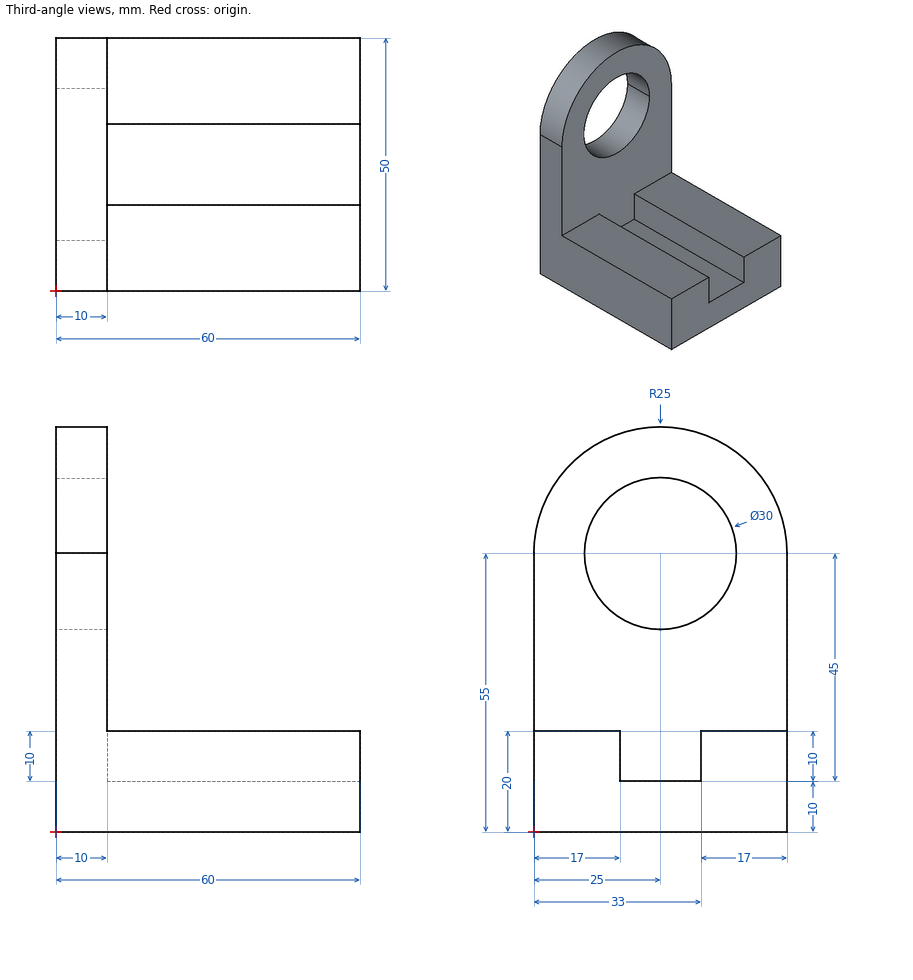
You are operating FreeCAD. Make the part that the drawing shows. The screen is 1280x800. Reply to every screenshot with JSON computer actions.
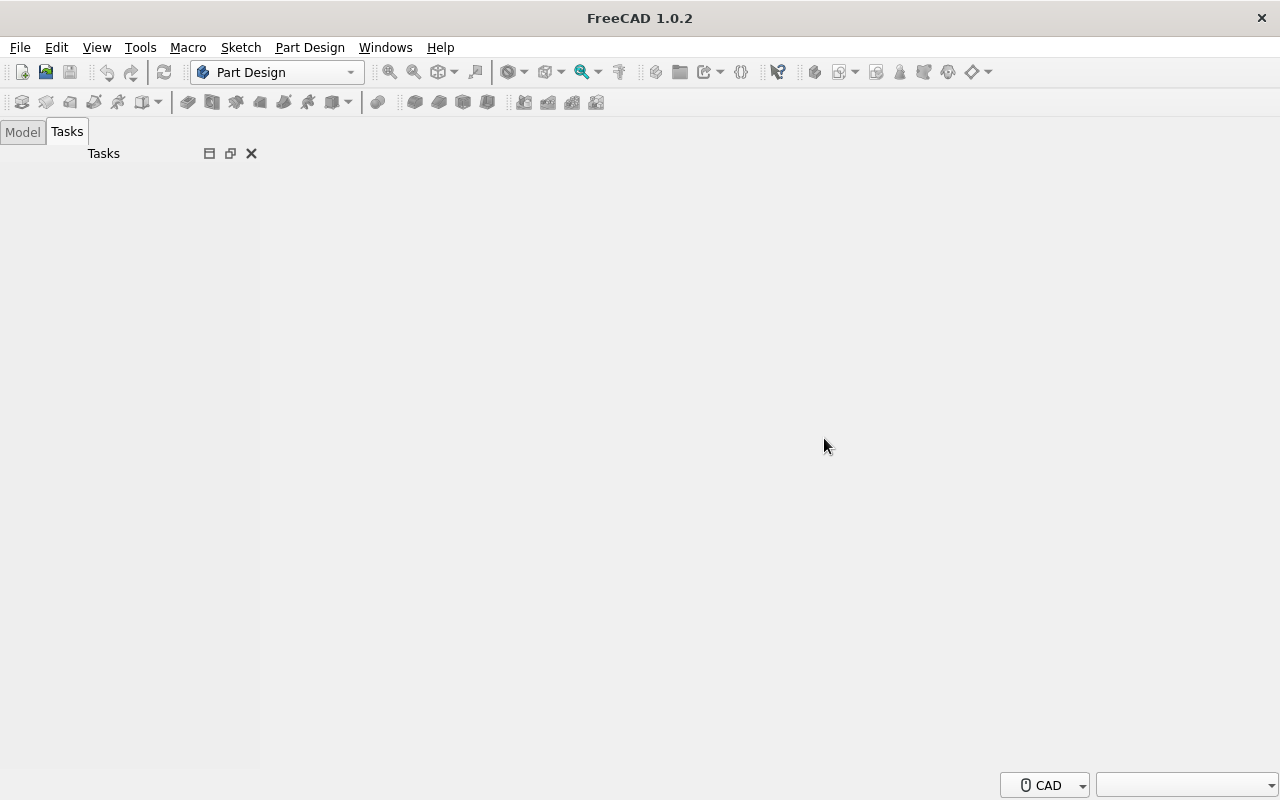
{"action": "left_click", "coordinate": [22, 72]}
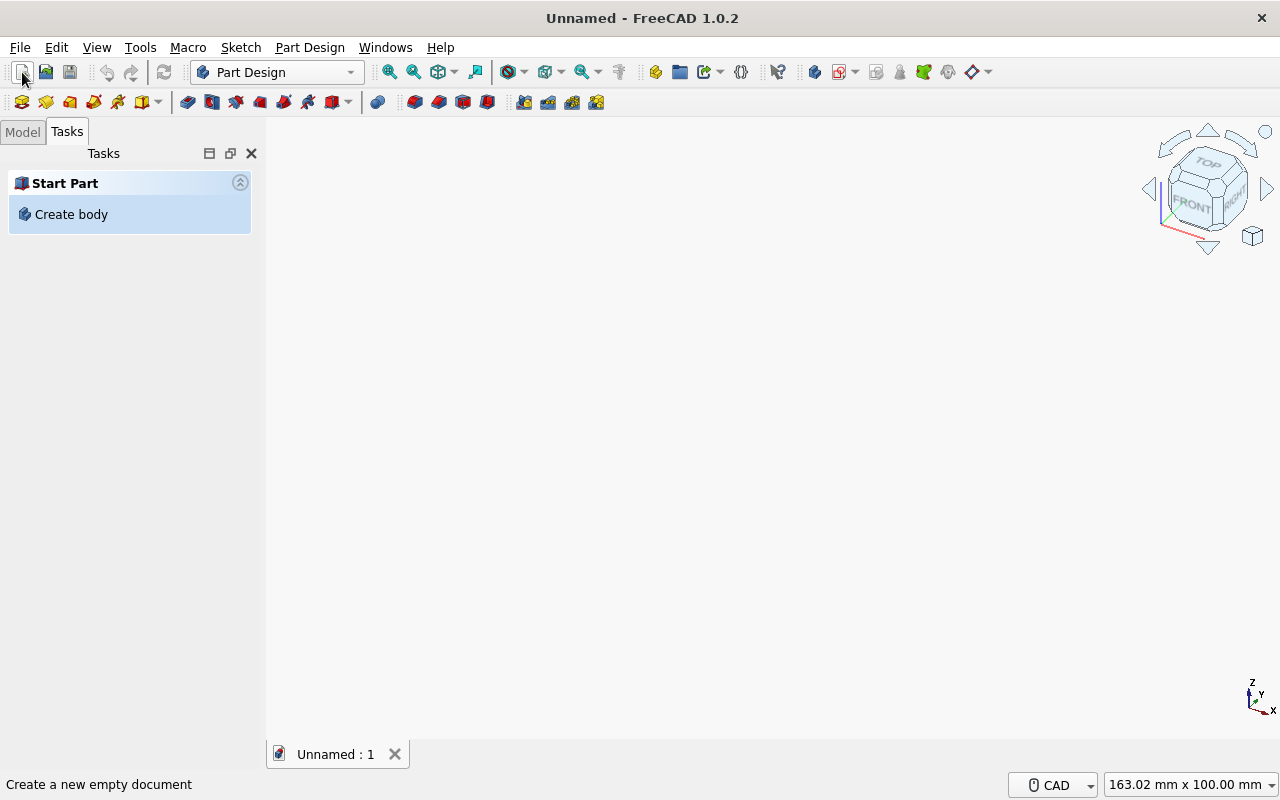
{"action": "left_click", "coordinate": [840, 72]}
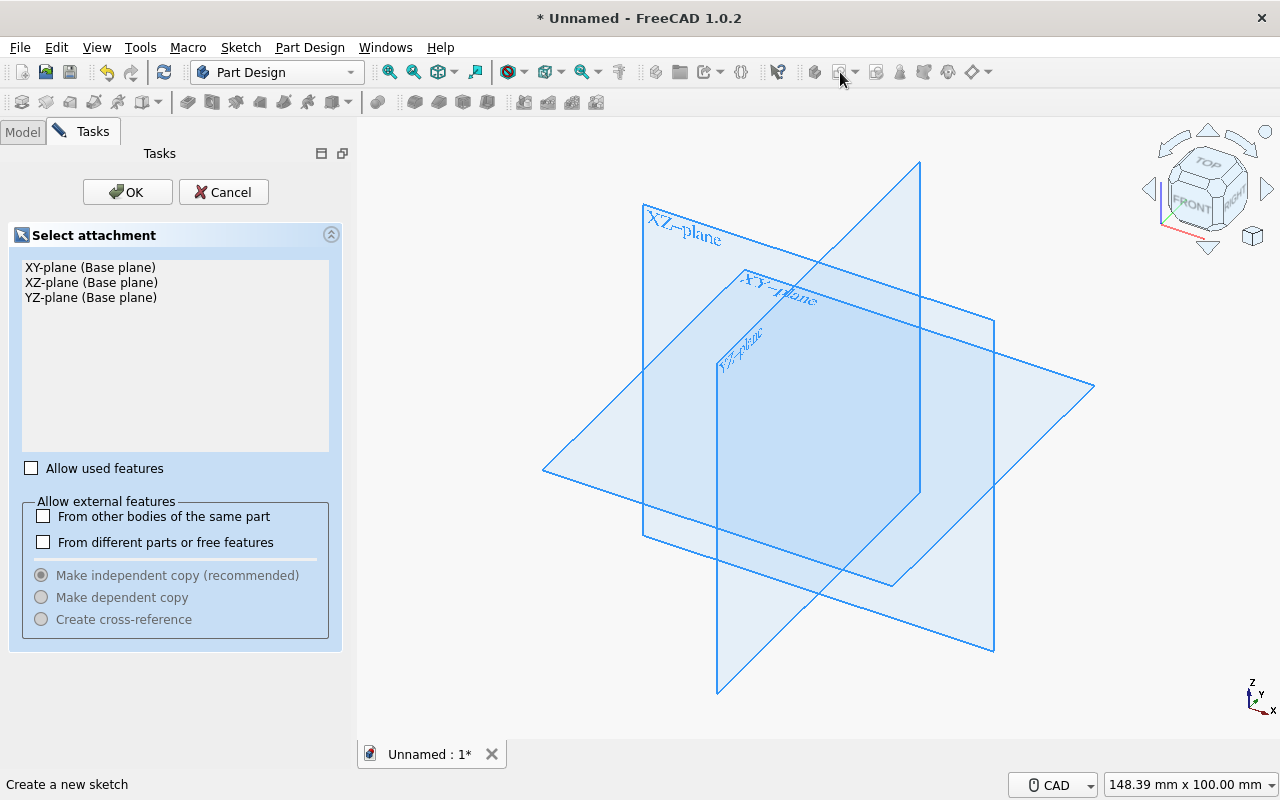
{"action": "left_click", "coordinate": [82, 268]}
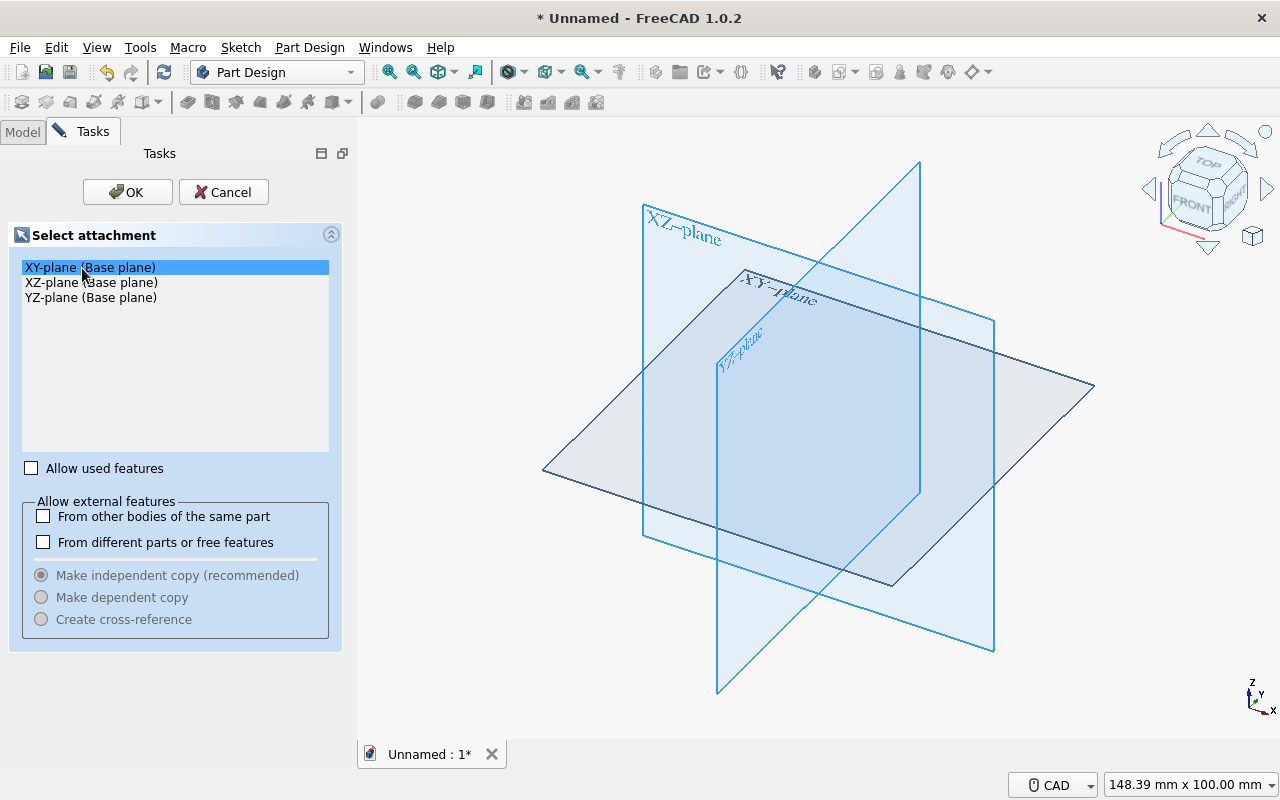
{"action": "left_click", "coordinate": [128, 192]}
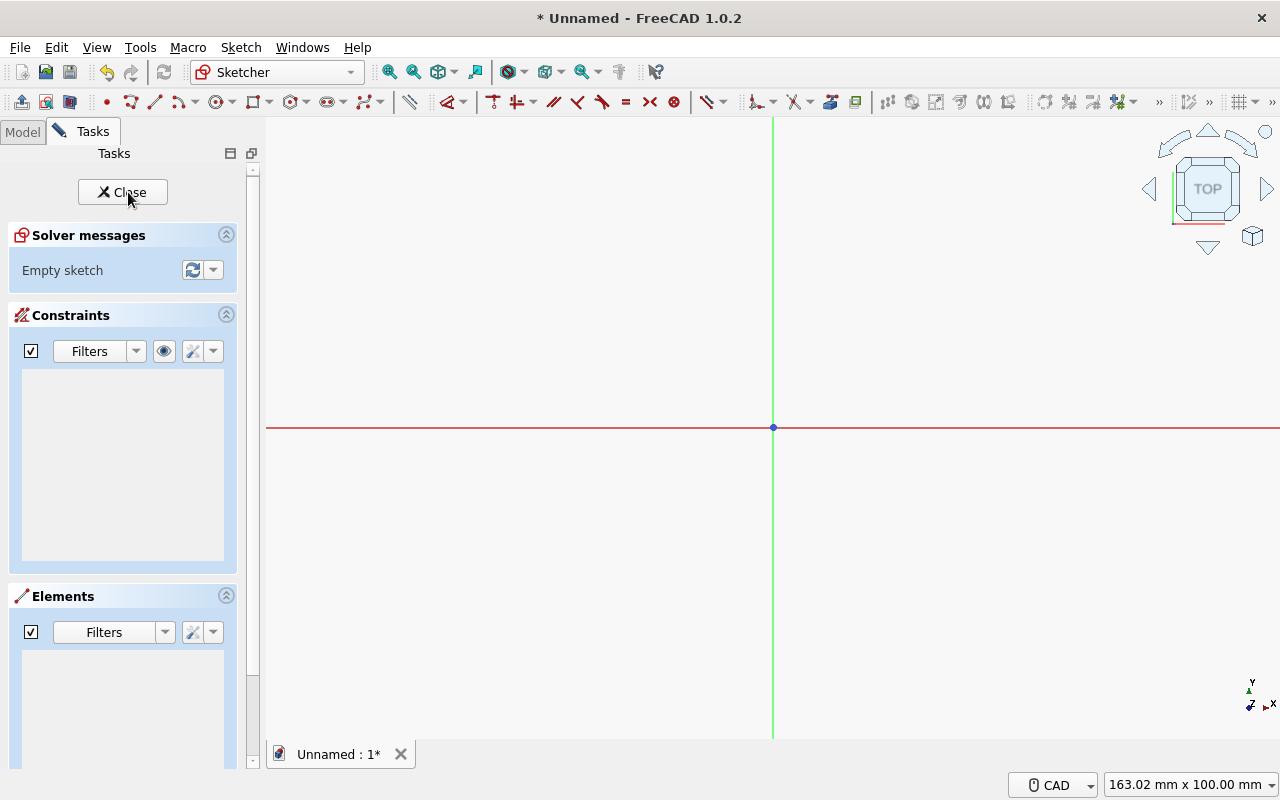
{"action": "scroll", "coordinate": [294, 711], "scroll_direction": "down", "scroll_amount": 1}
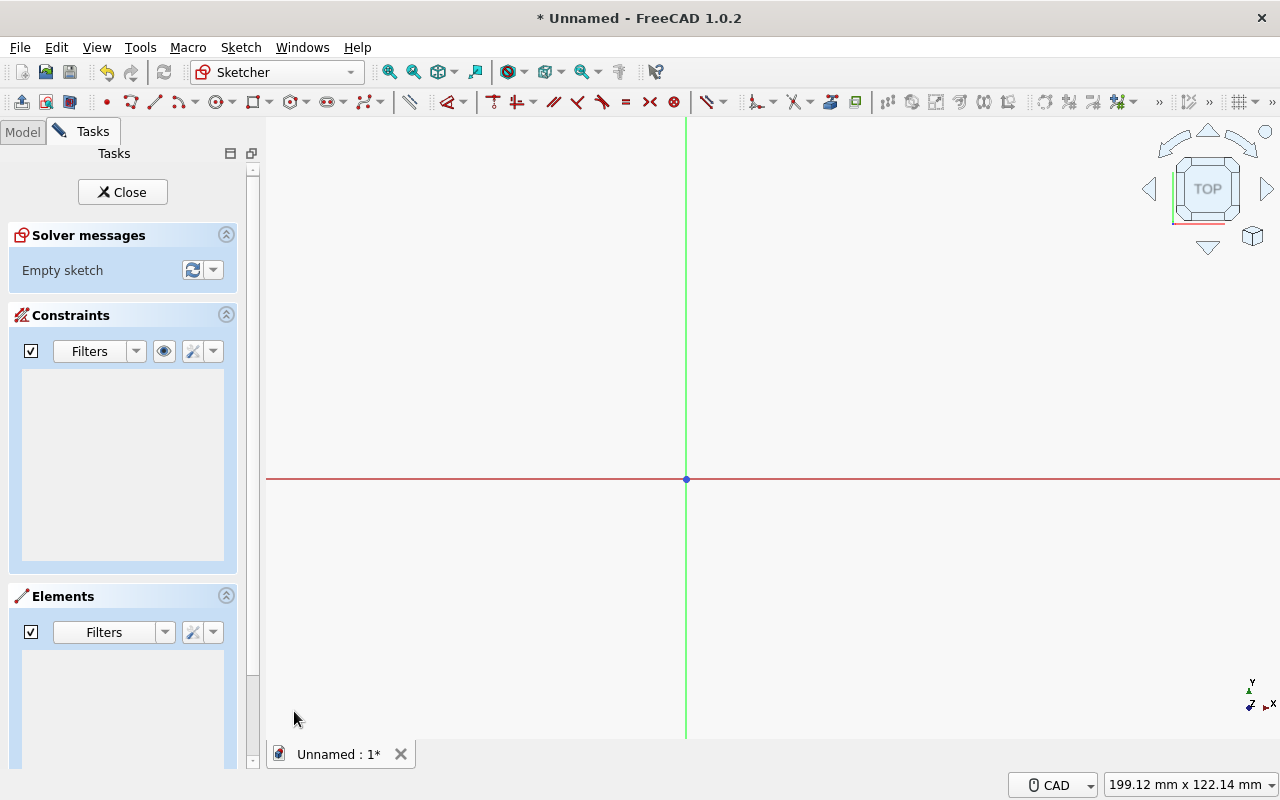
{"action": "scroll", "coordinate": [1112, 198], "scroll_direction": "up", "scroll_amount": 2}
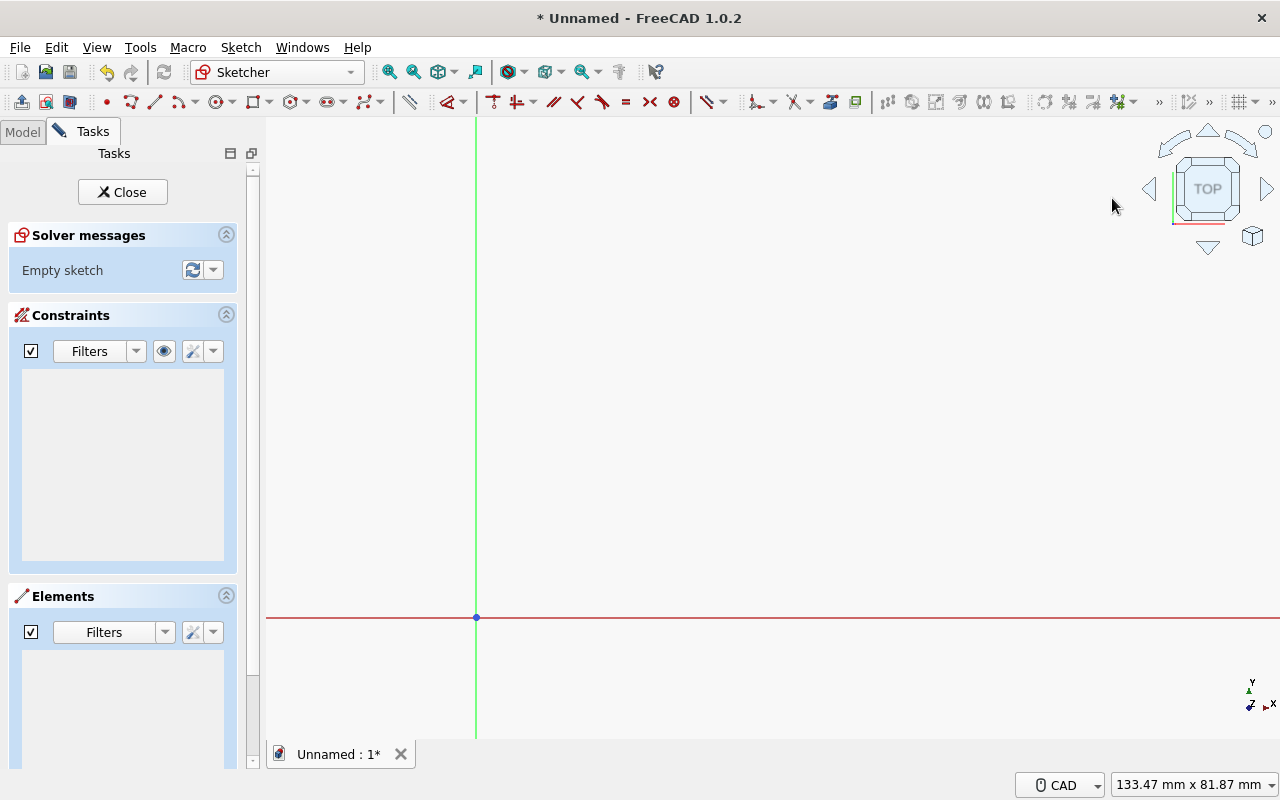
{"action": "left_click", "coordinate": [254, 102]}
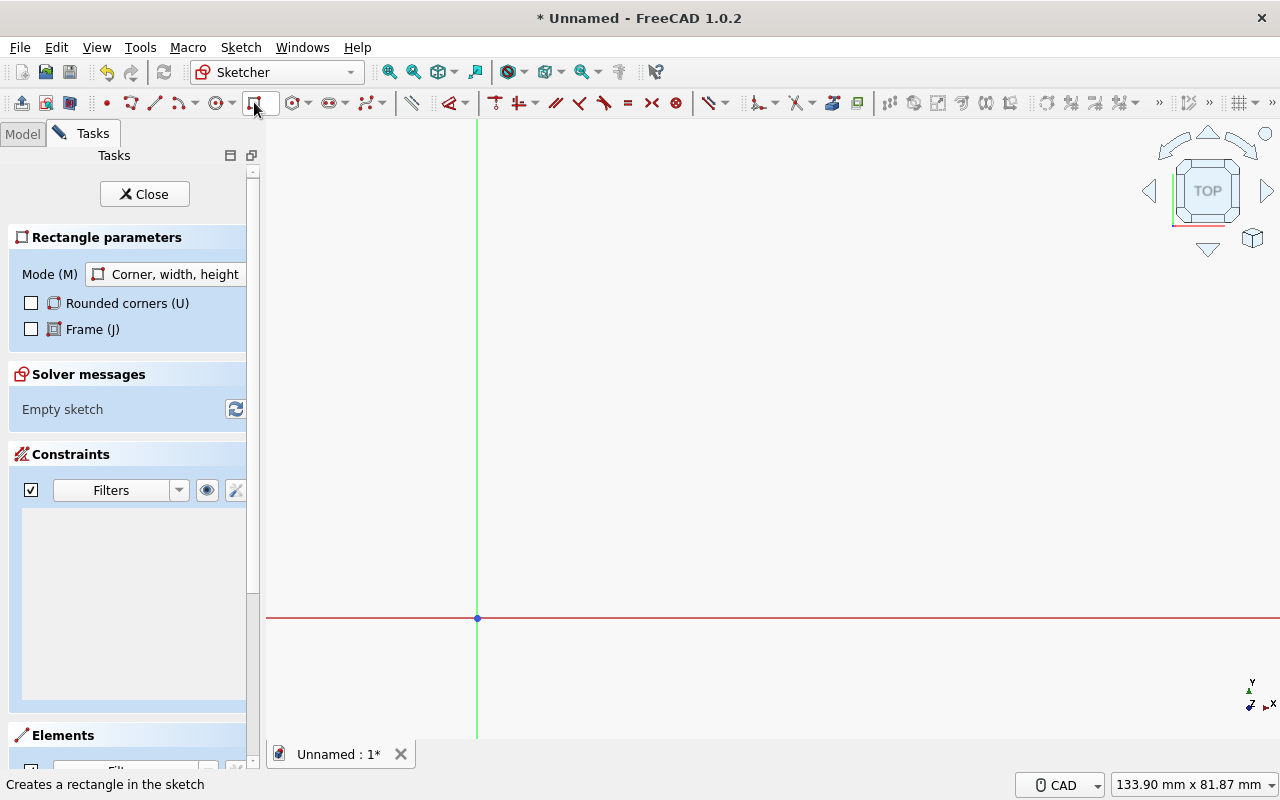
{"action": "left_click", "coordinate": [477, 618]}
{"action": "left_click", "coordinate": [932, 240]}
{"action": "key", "text": "Escape"}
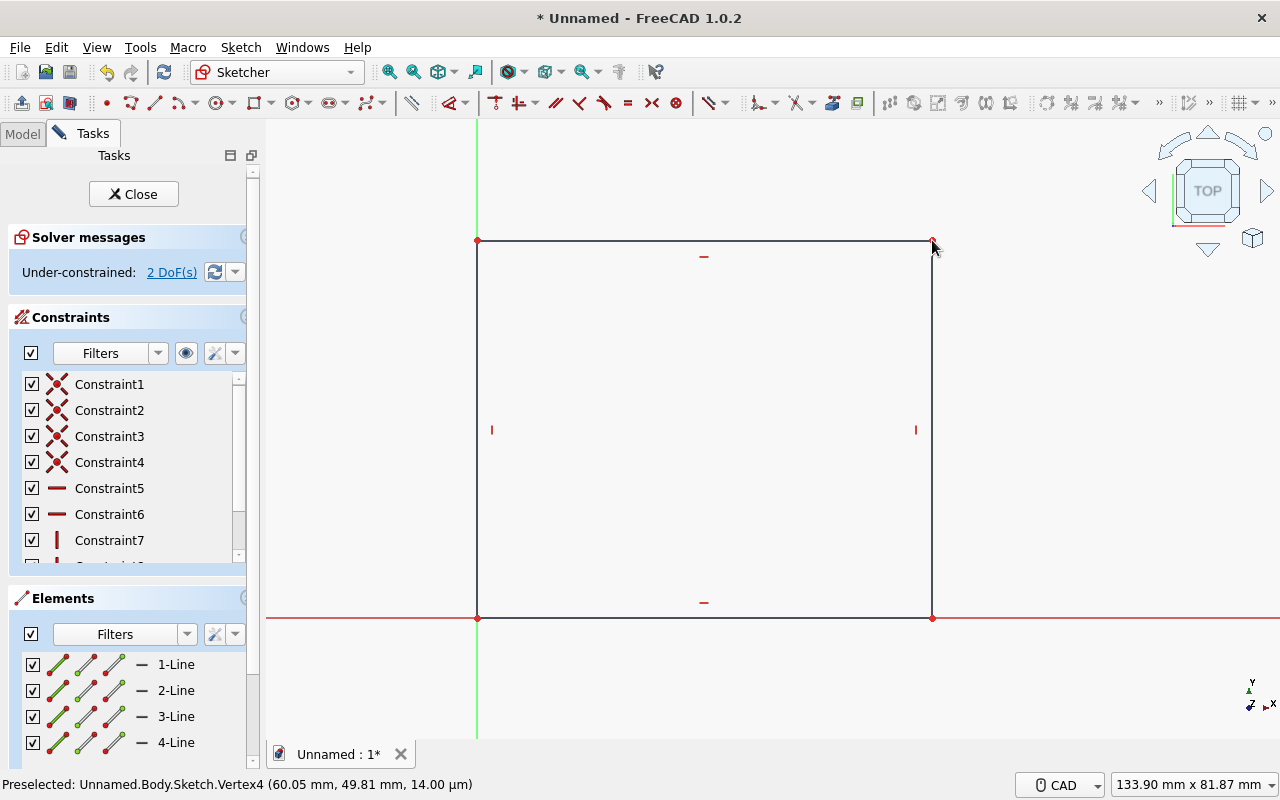
{"action": "left_click", "coordinate": [614, 618]}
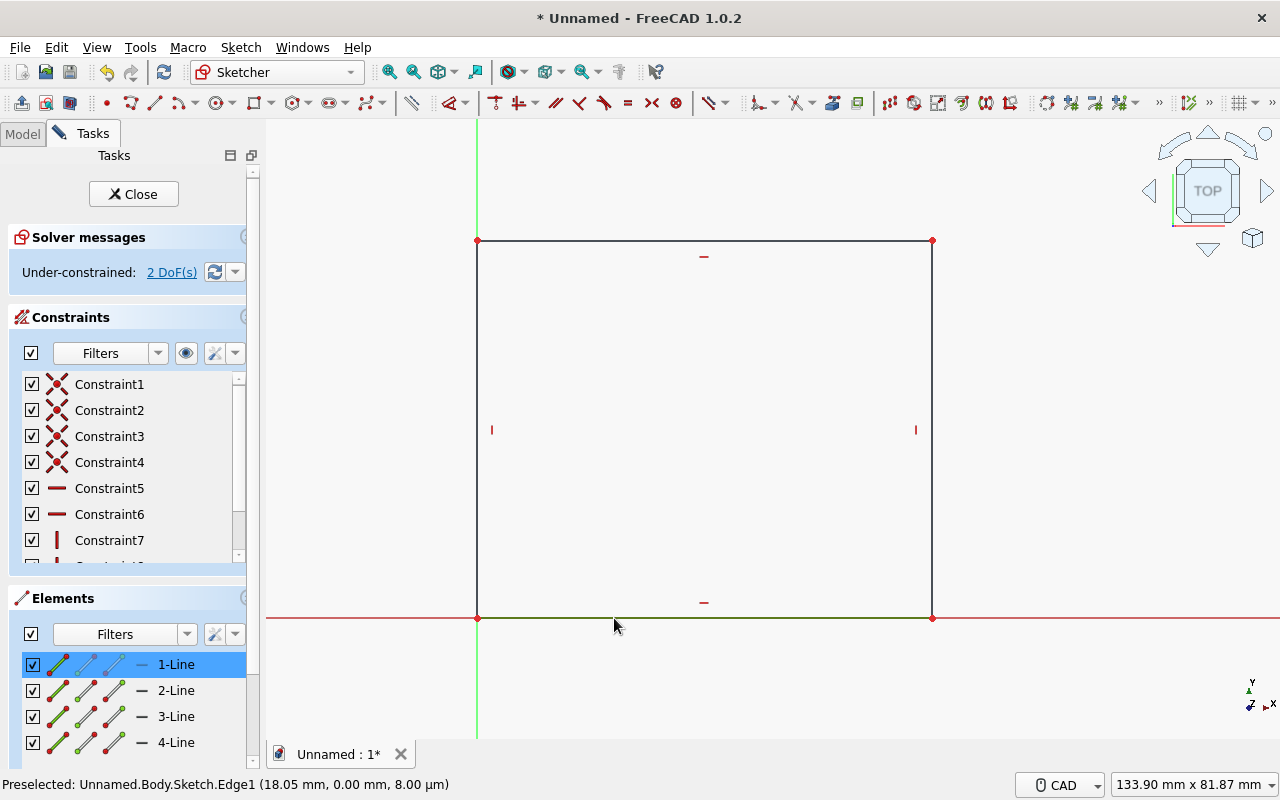
{"action": "left_click", "coordinate": [468, 104]}